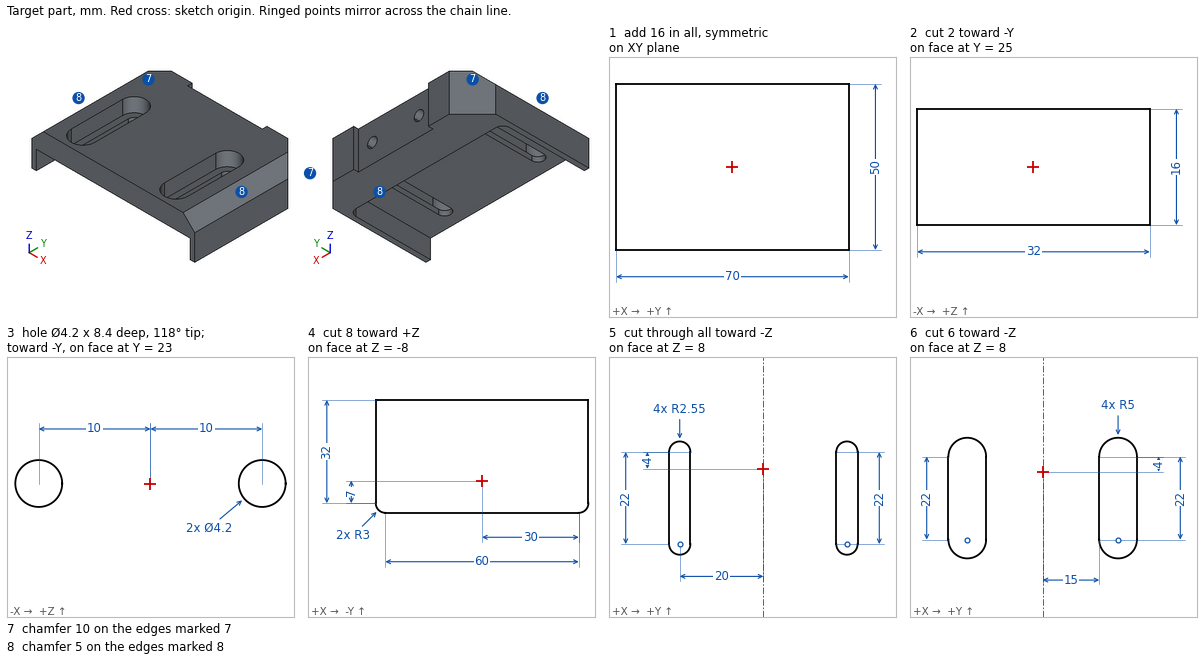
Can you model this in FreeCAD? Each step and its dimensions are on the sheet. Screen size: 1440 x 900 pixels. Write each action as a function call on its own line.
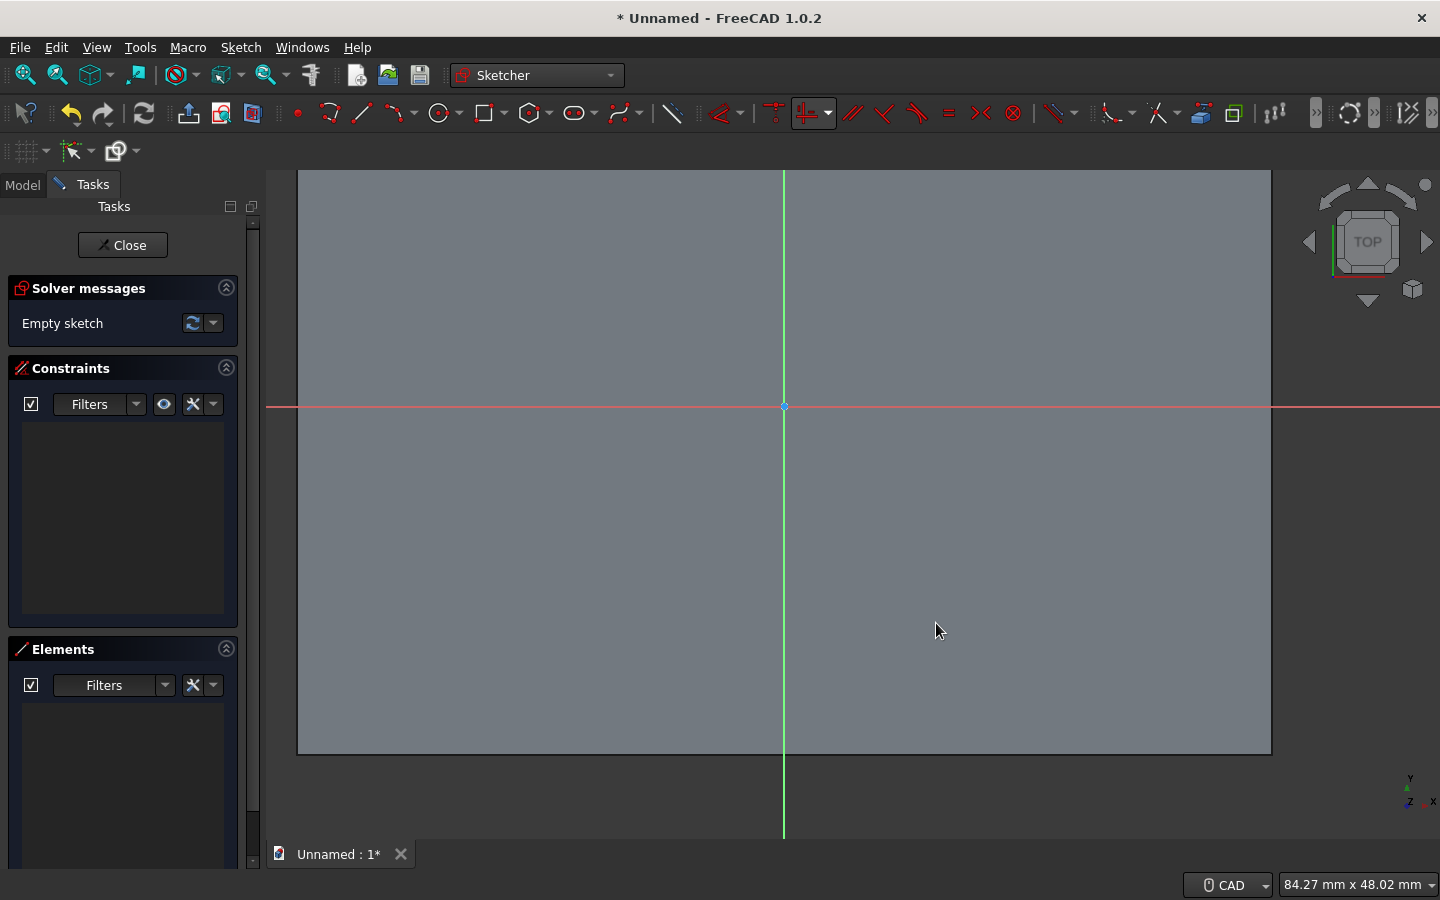
click(574, 114)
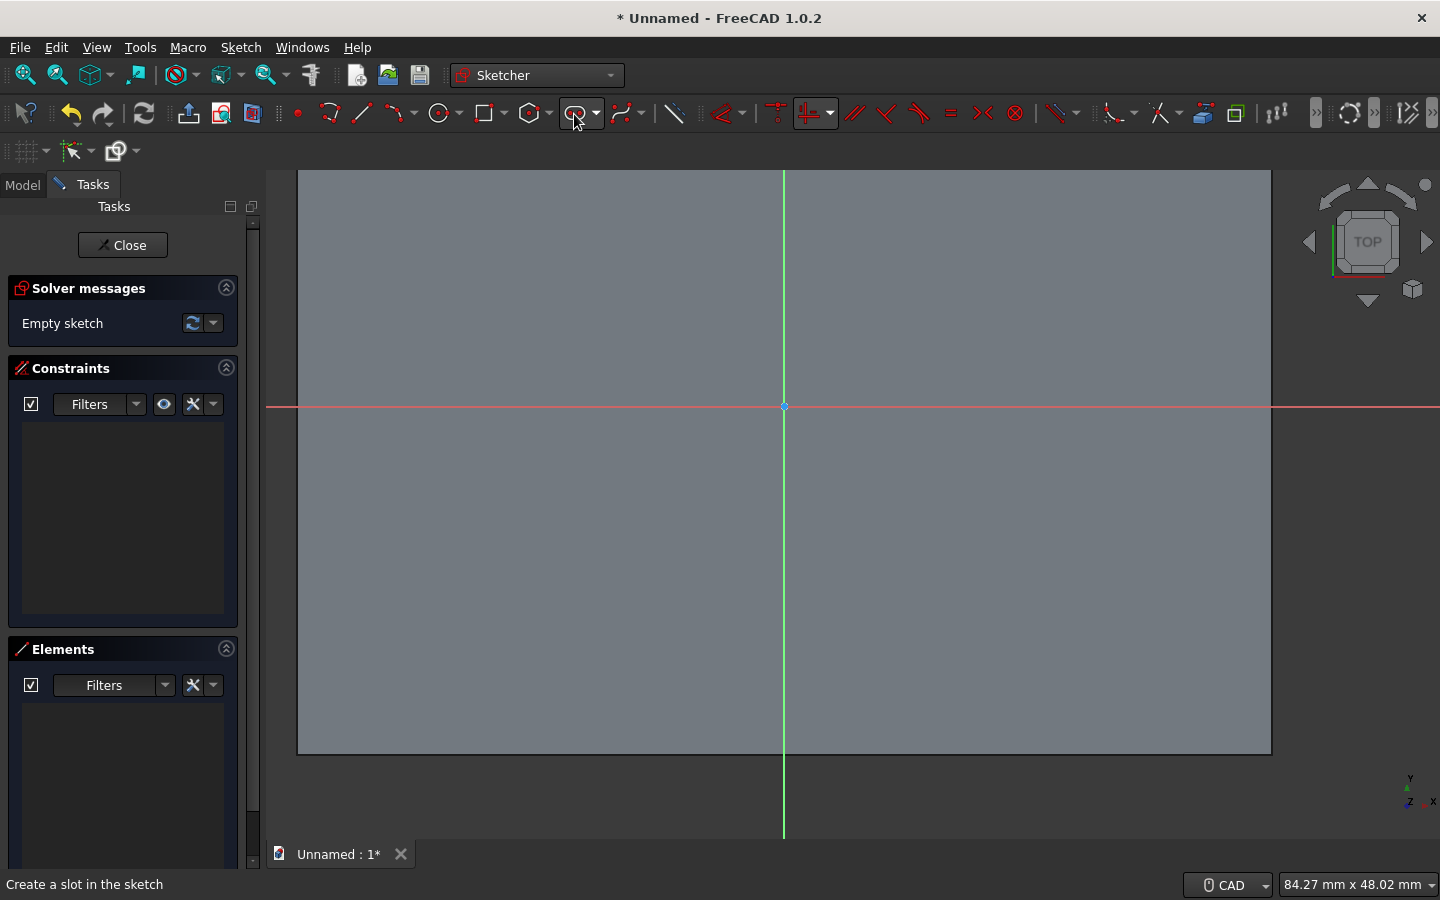
click(506, 657)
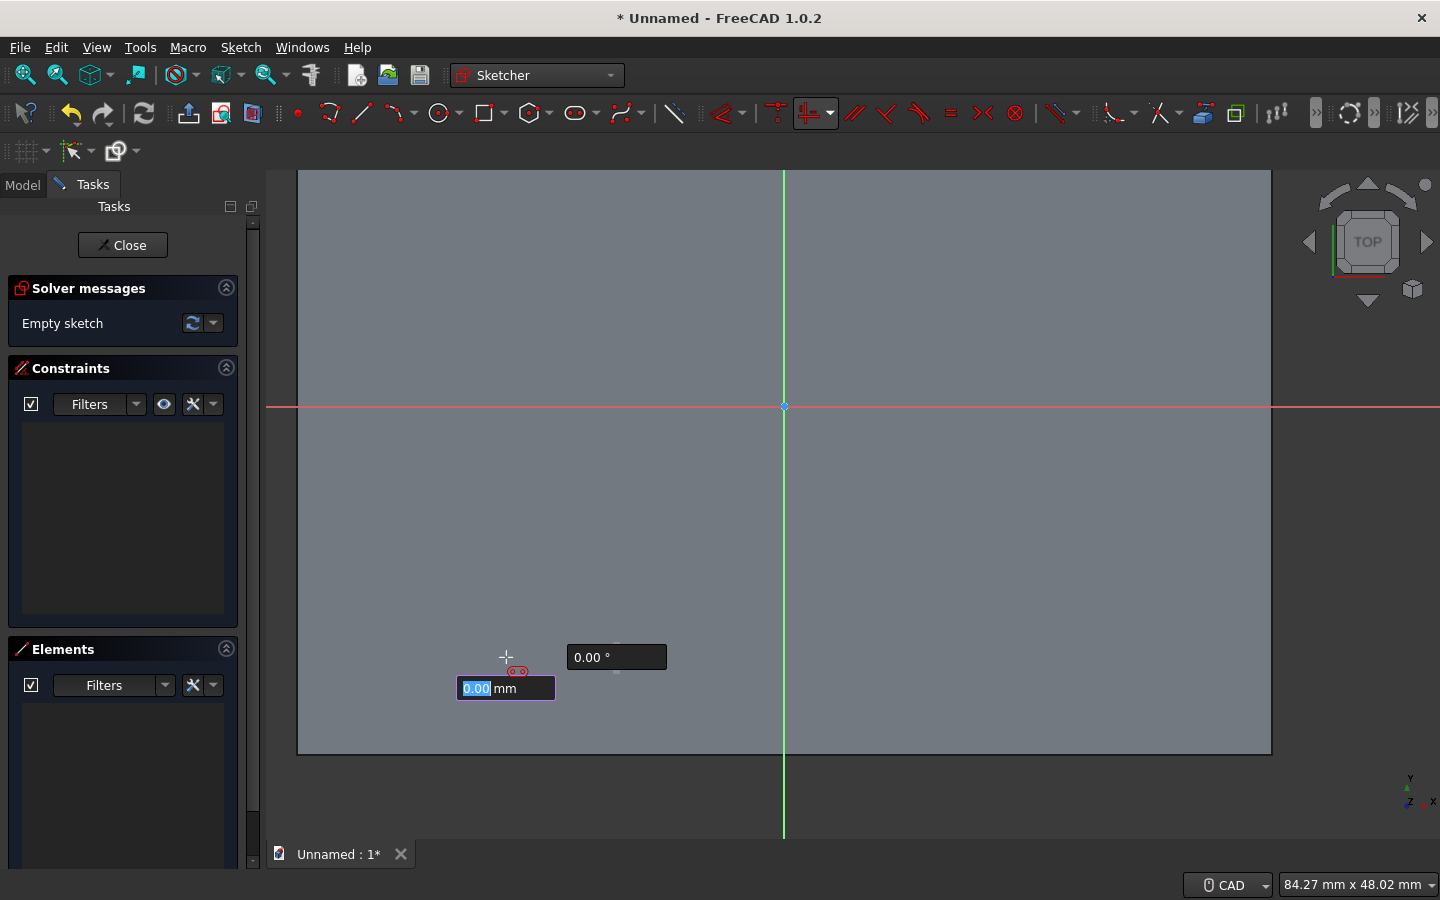
click(506, 351)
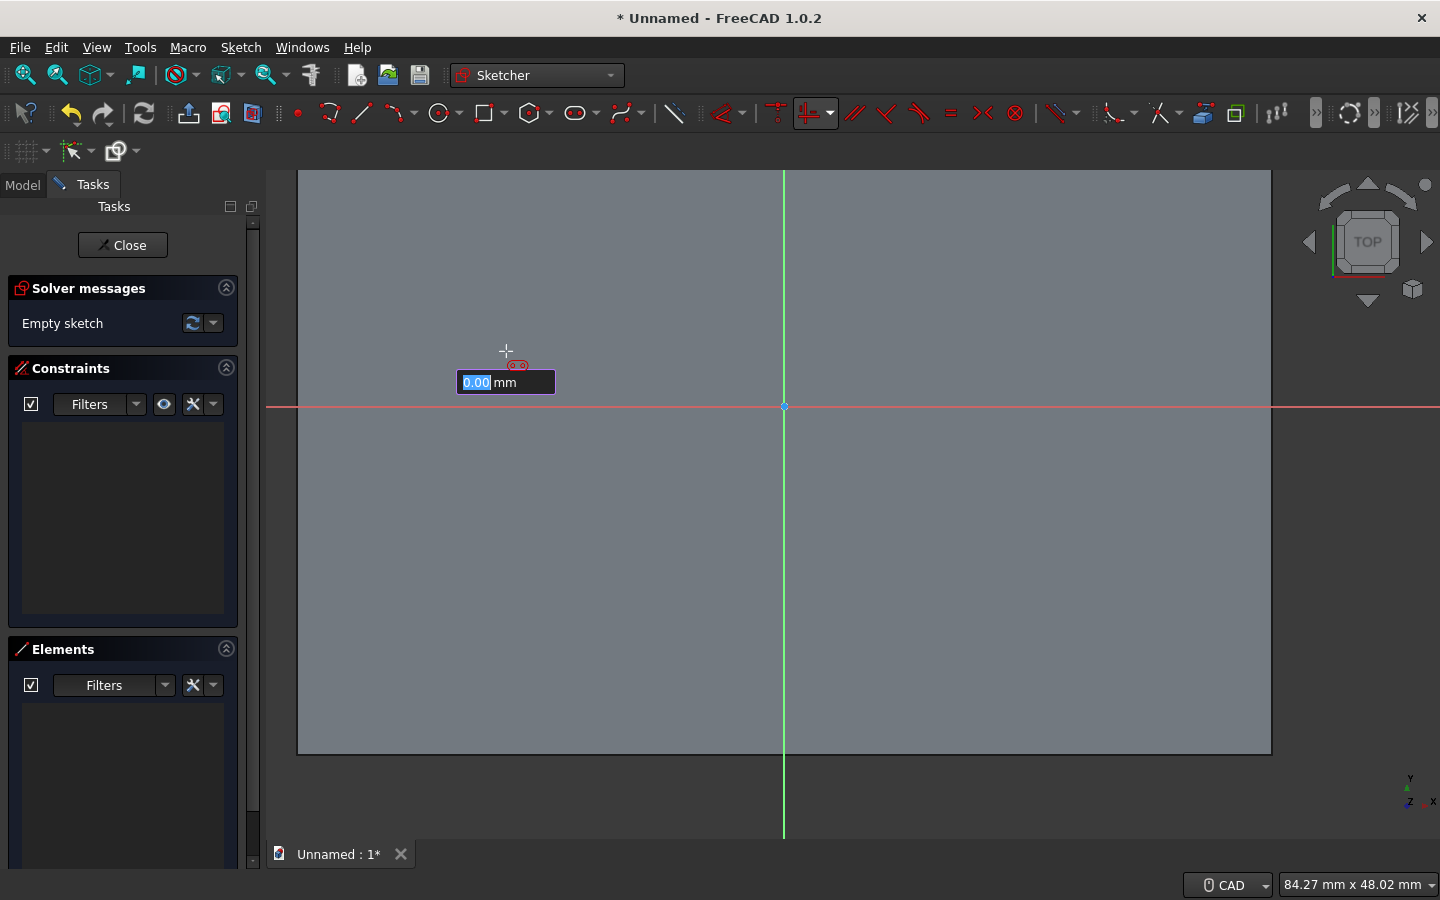
click(470, 504)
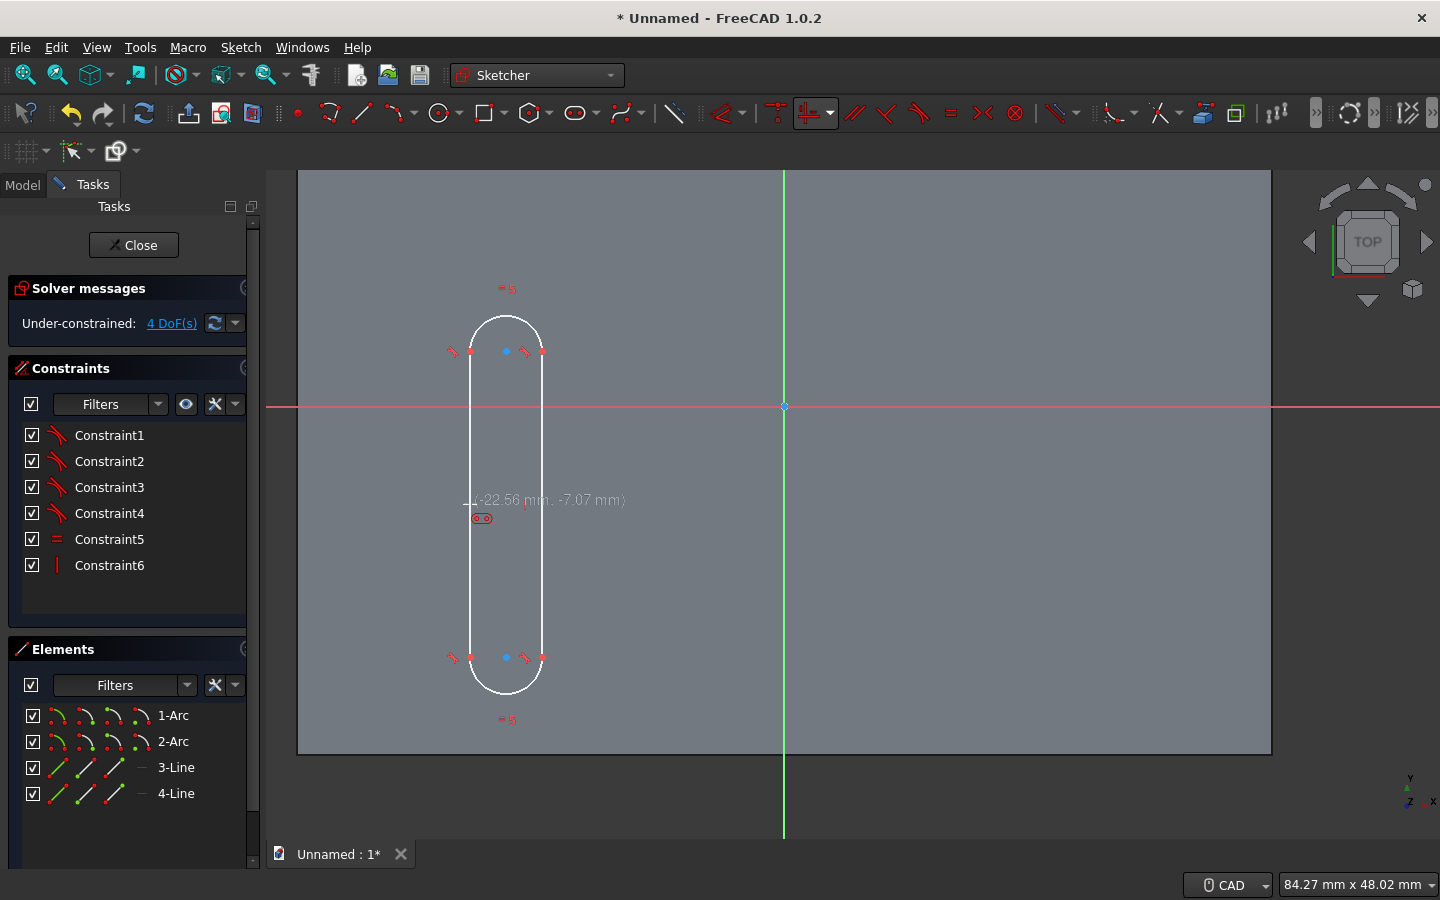
click(1063, 657)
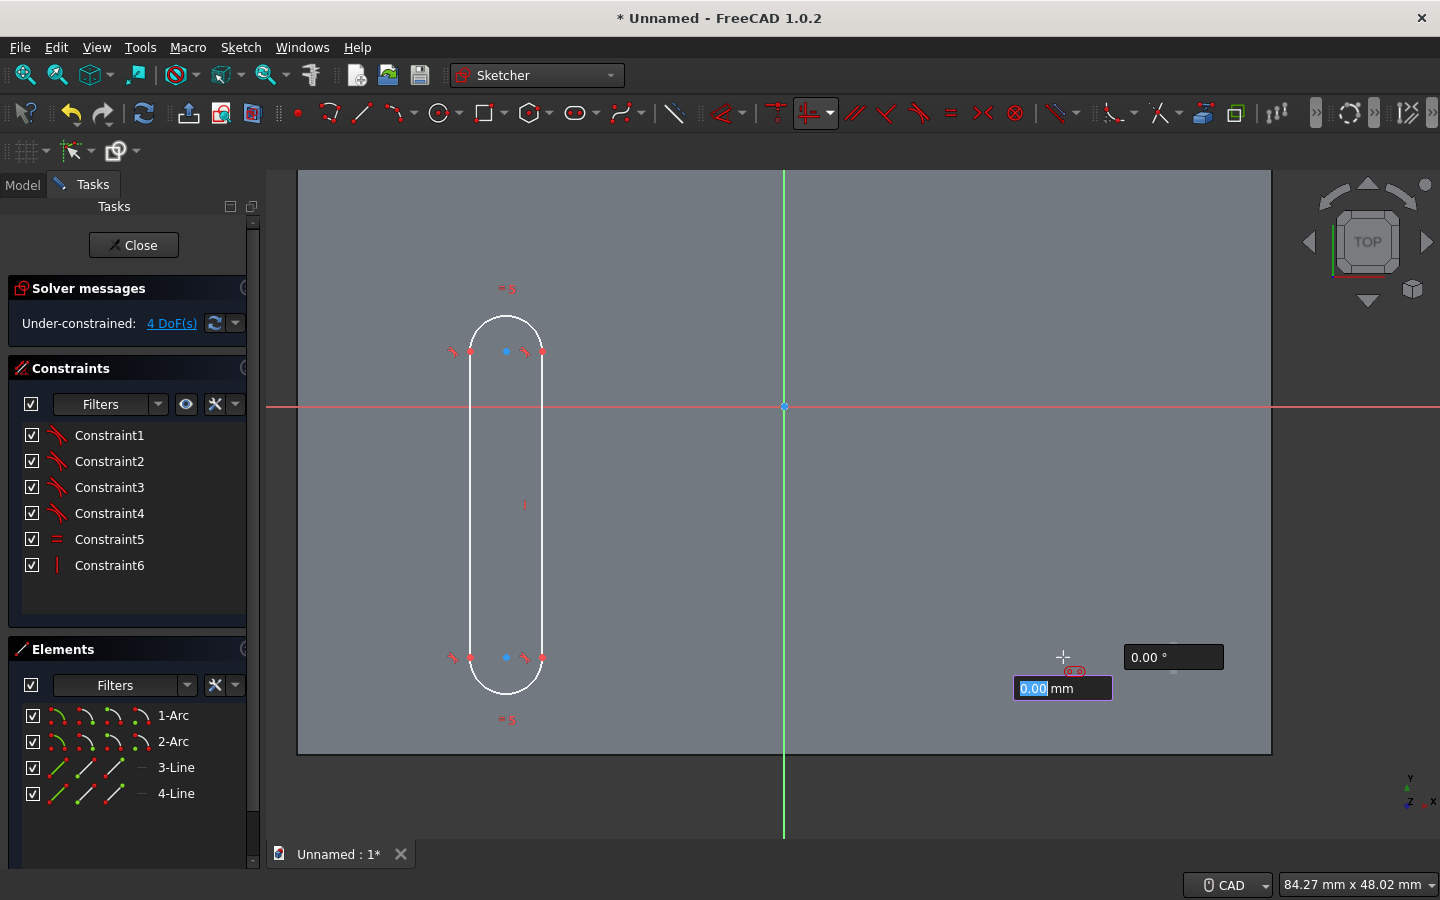
click(1063, 351)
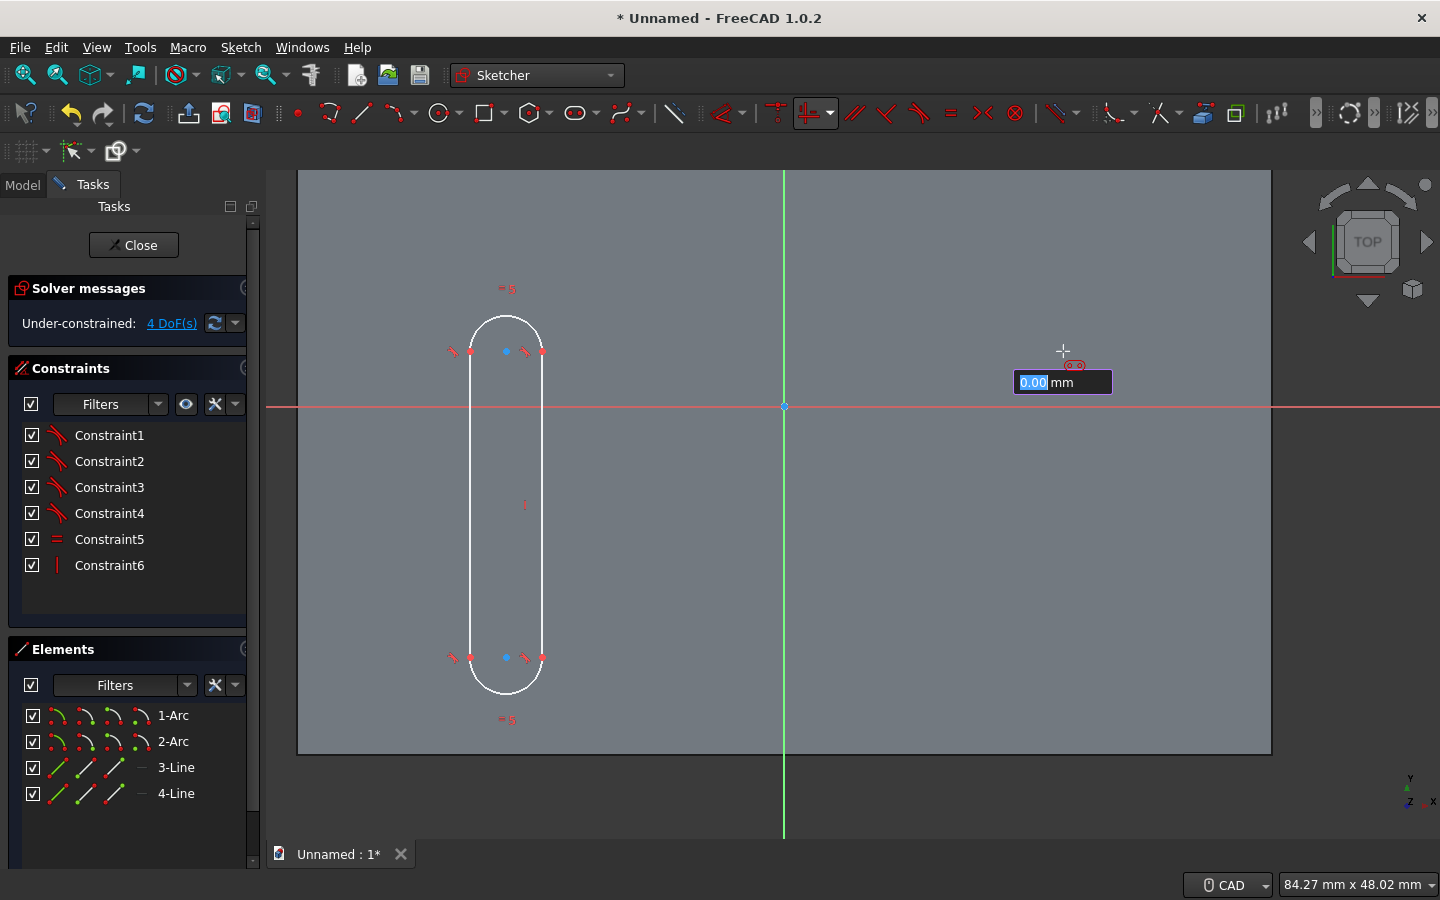
click(1027, 504)
key(Escape)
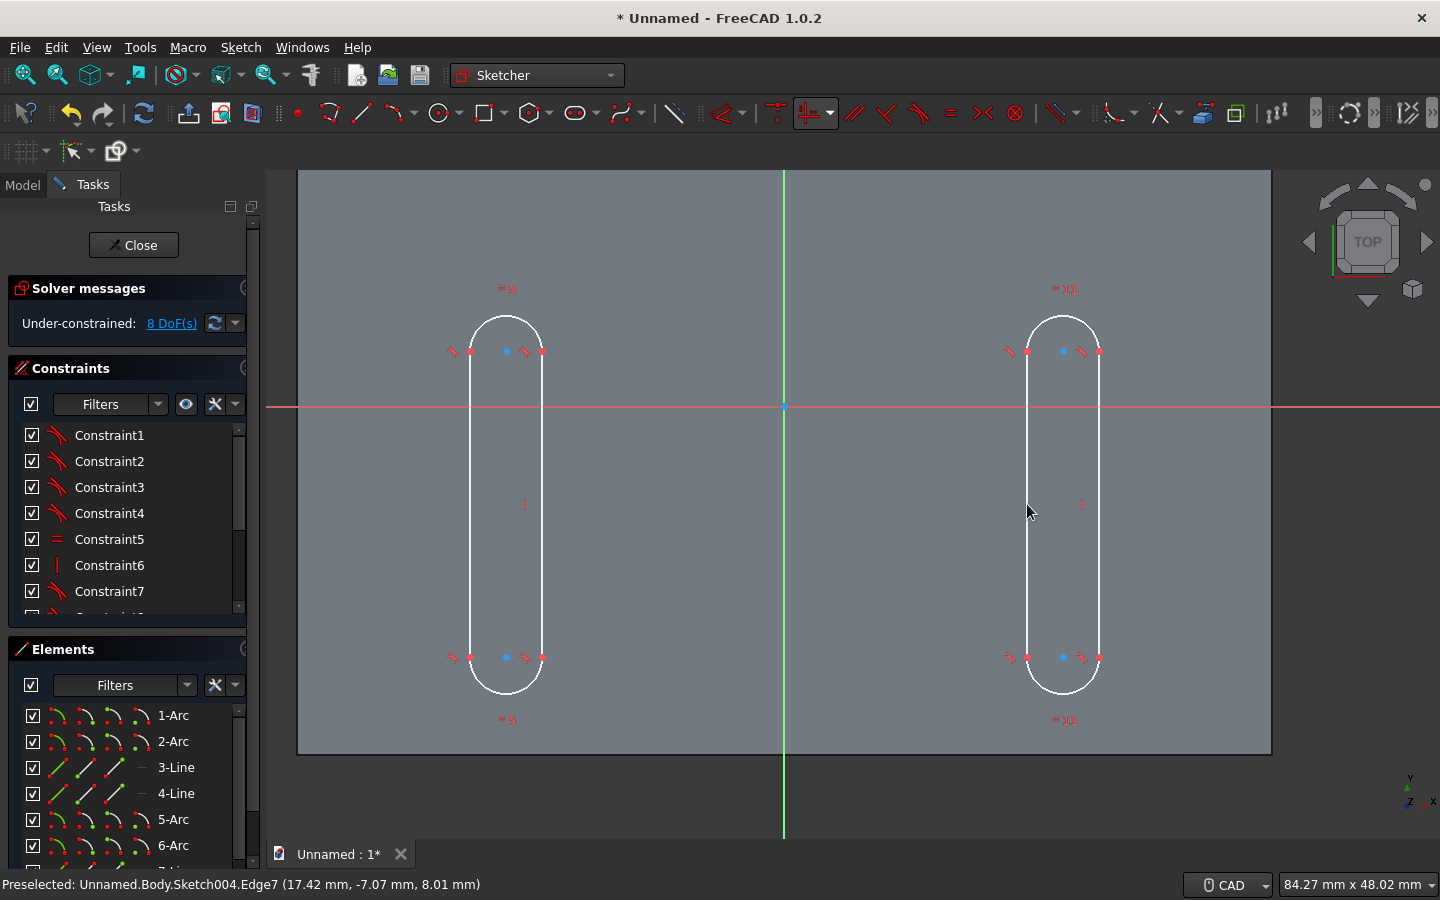
click(485, 687)